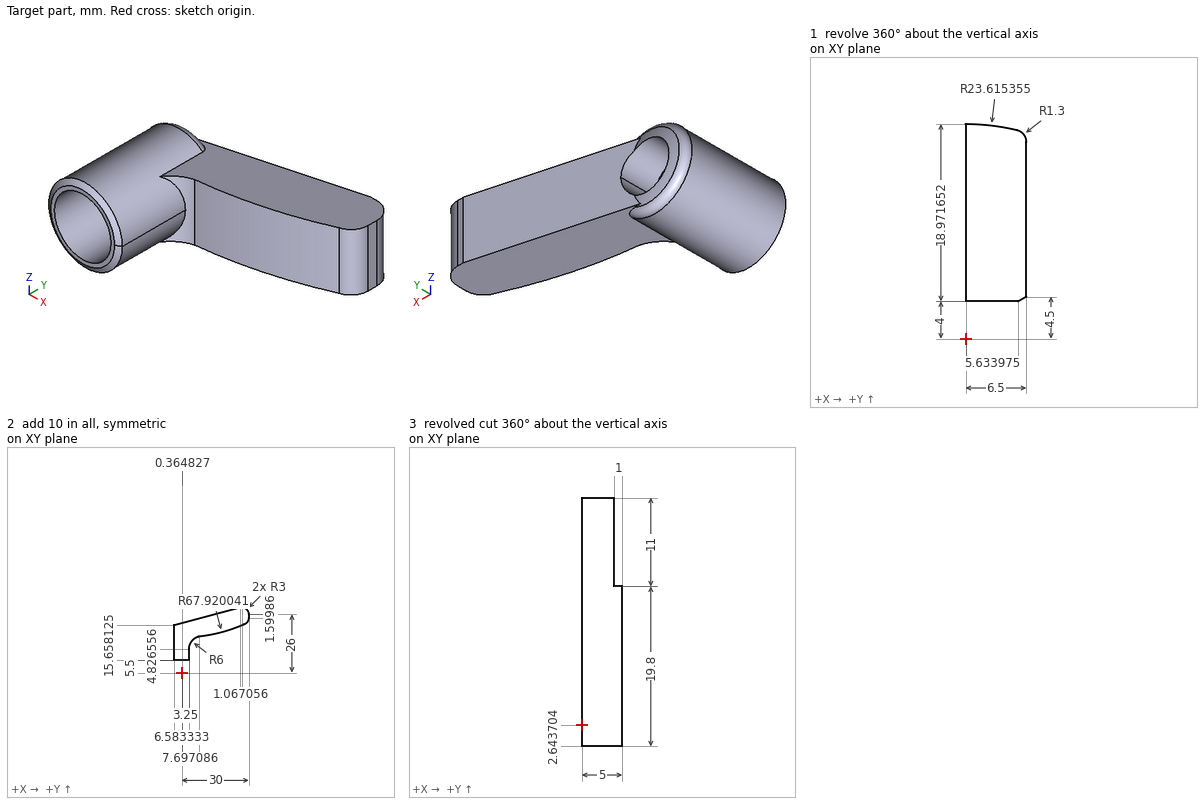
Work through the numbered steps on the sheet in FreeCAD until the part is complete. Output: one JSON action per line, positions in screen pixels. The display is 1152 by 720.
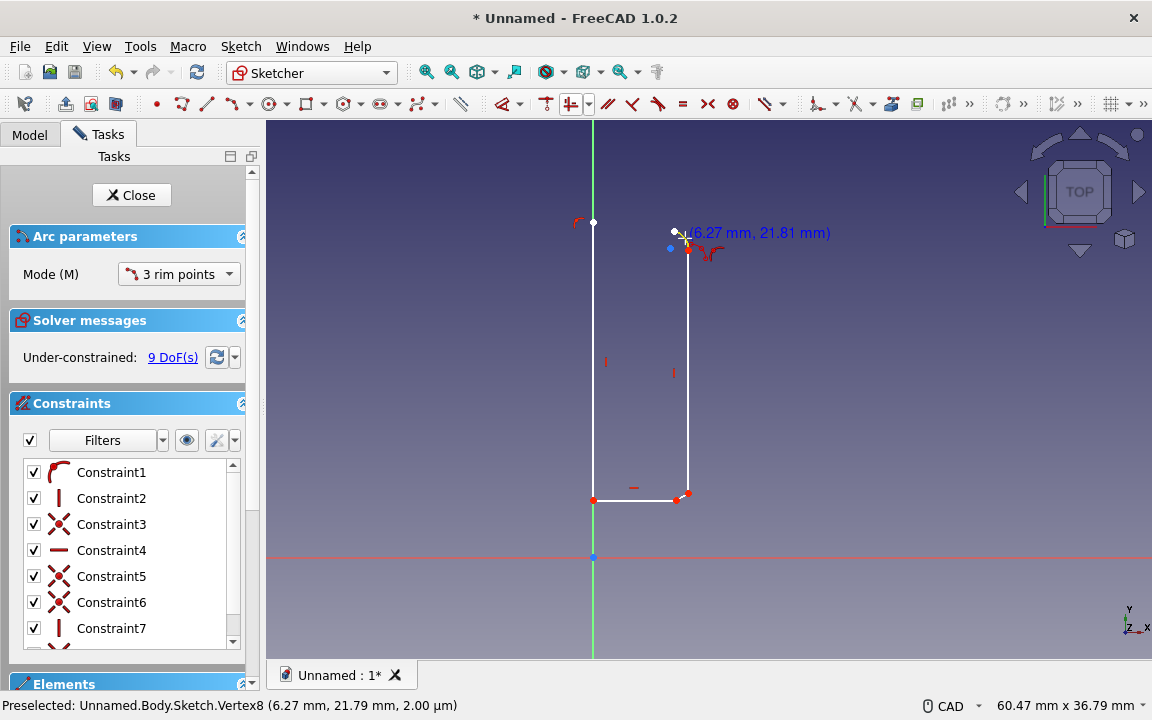
{"action": "left_click", "coordinate": [674, 232]}
{"action": "left_click", "coordinate": [593, 223]}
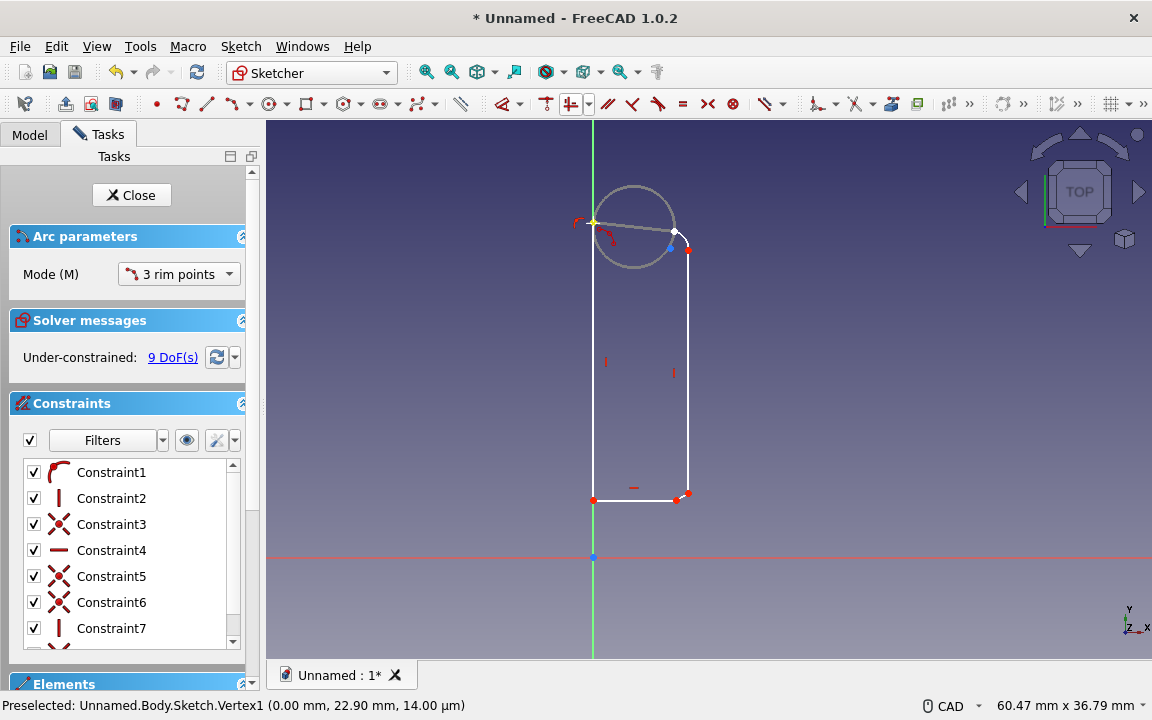
{"action": "scroll", "coordinate": [634, 224], "scroll_direction": "up", "scroll_amount": 10}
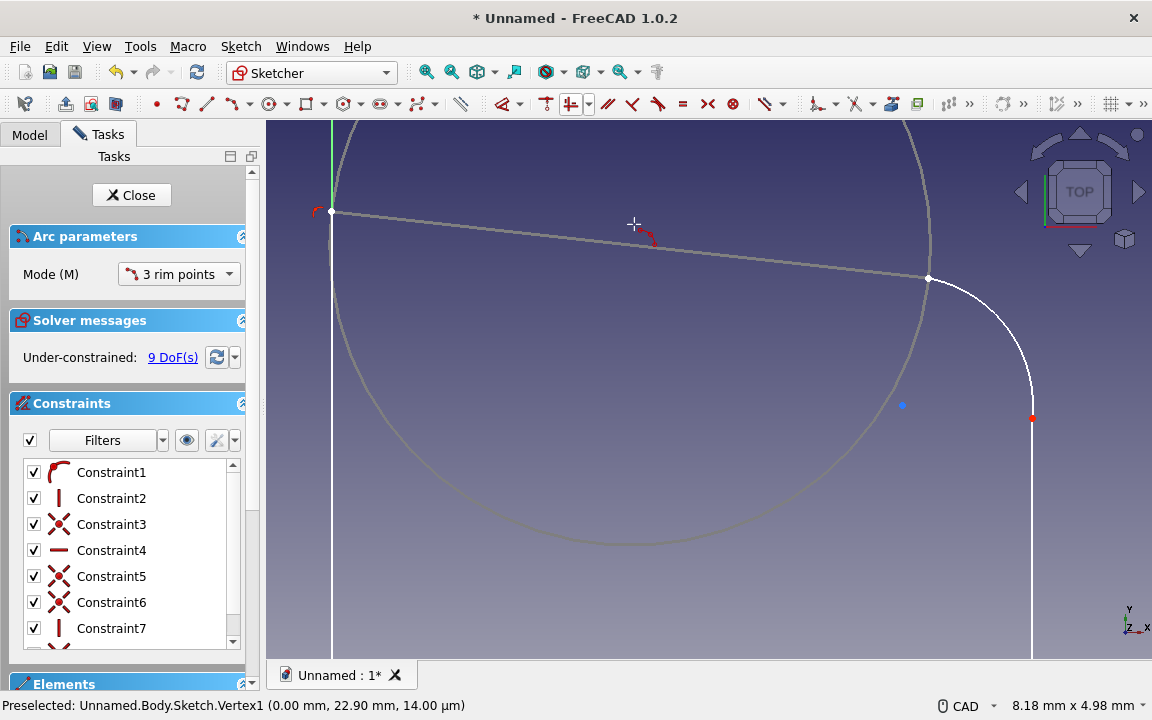
{"action": "left_click", "coordinate": [631, 221]}
{"action": "key", "text": "Escape"}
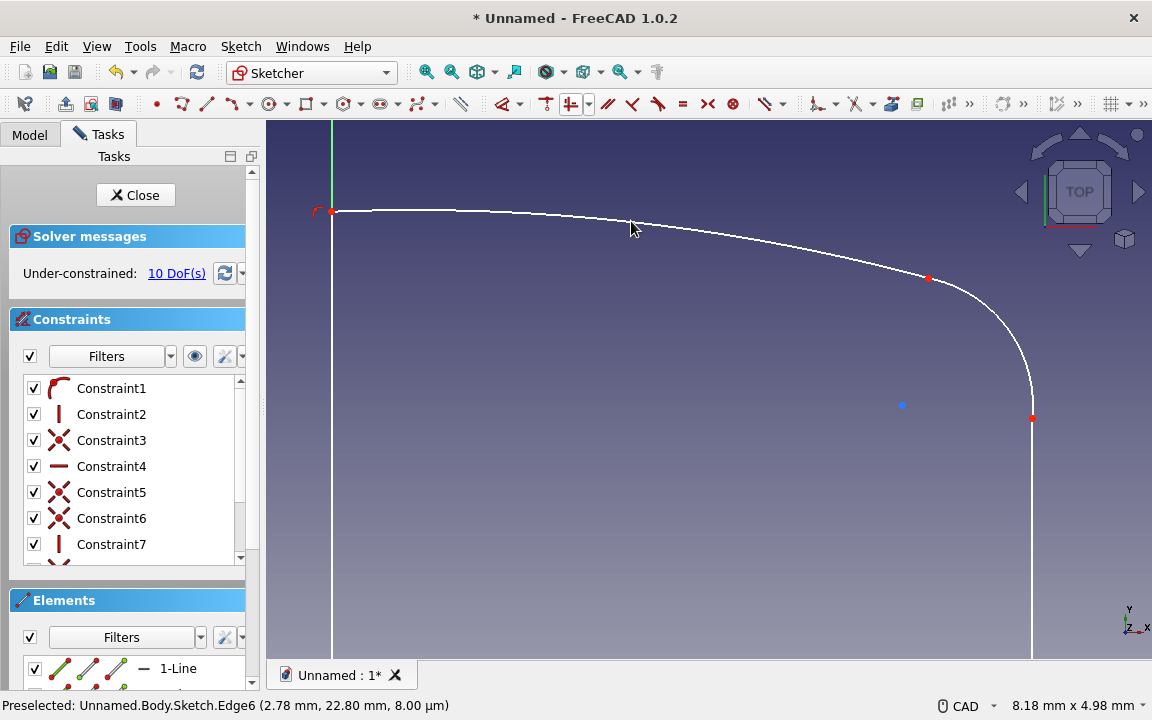
{"action": "scroll", "coordinate": [634, 224], "scroll_direction": "down", "scroll_amount": 10}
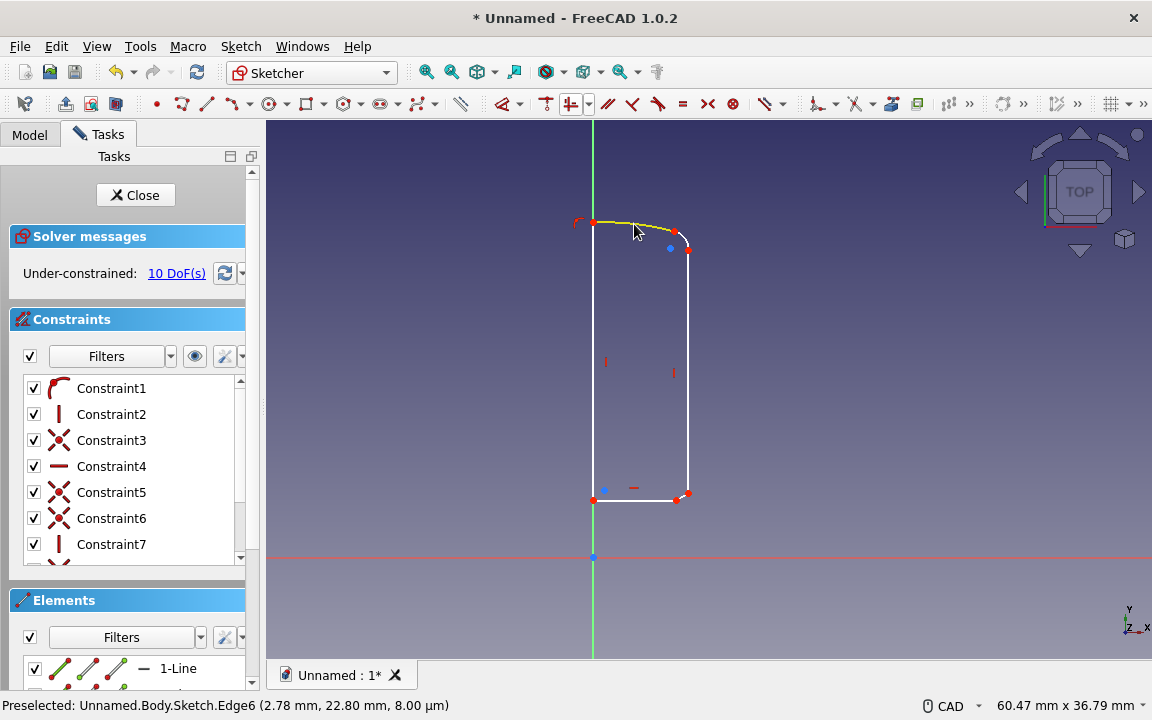
{"action": "left_click", "coordinate": [688, 421]}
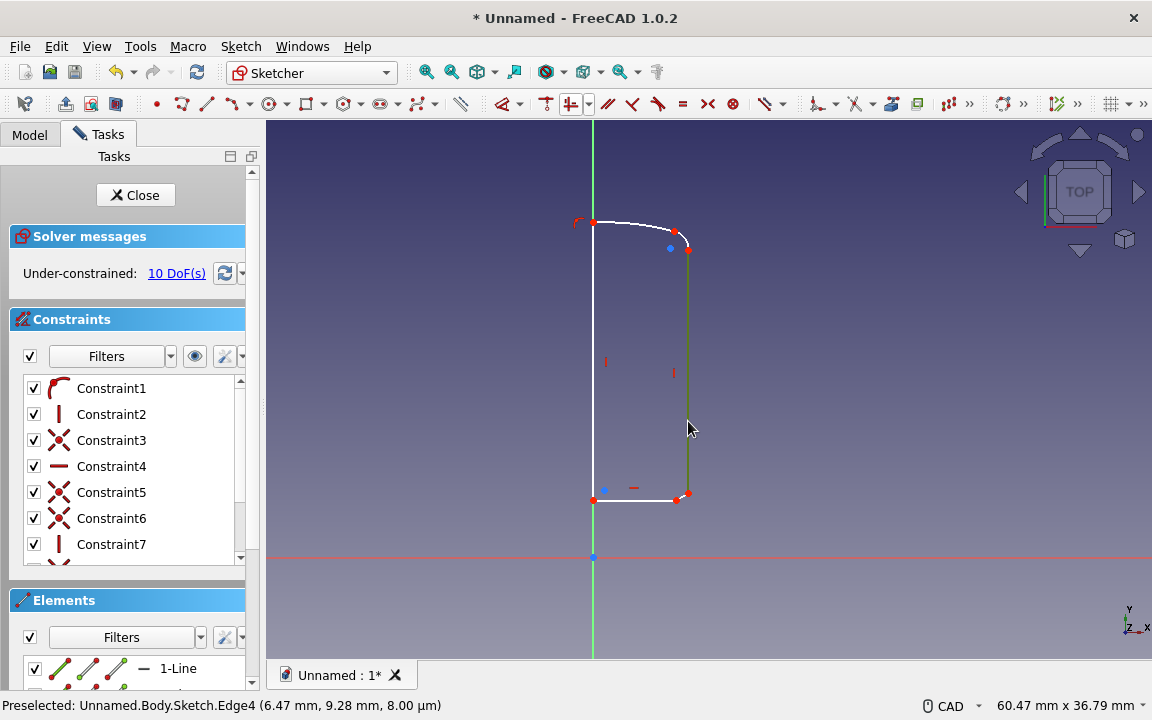
{"action": "left_click", "coordinate": [685, 238]}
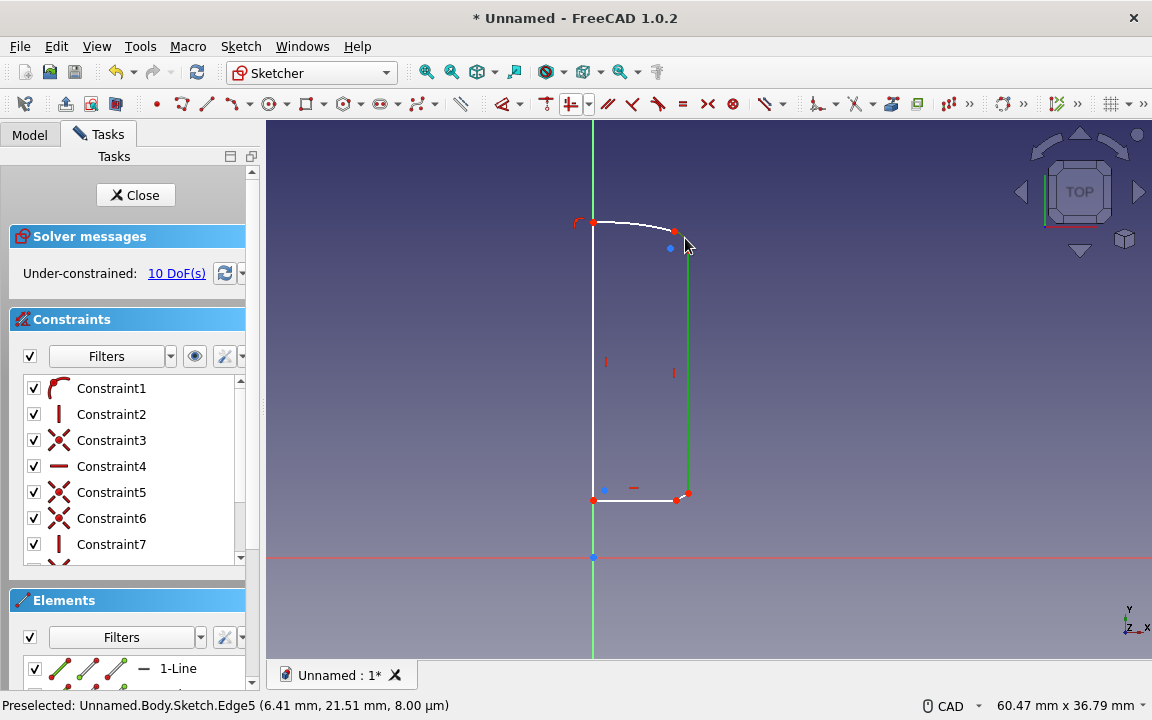
{"action": "key", "text": "t"}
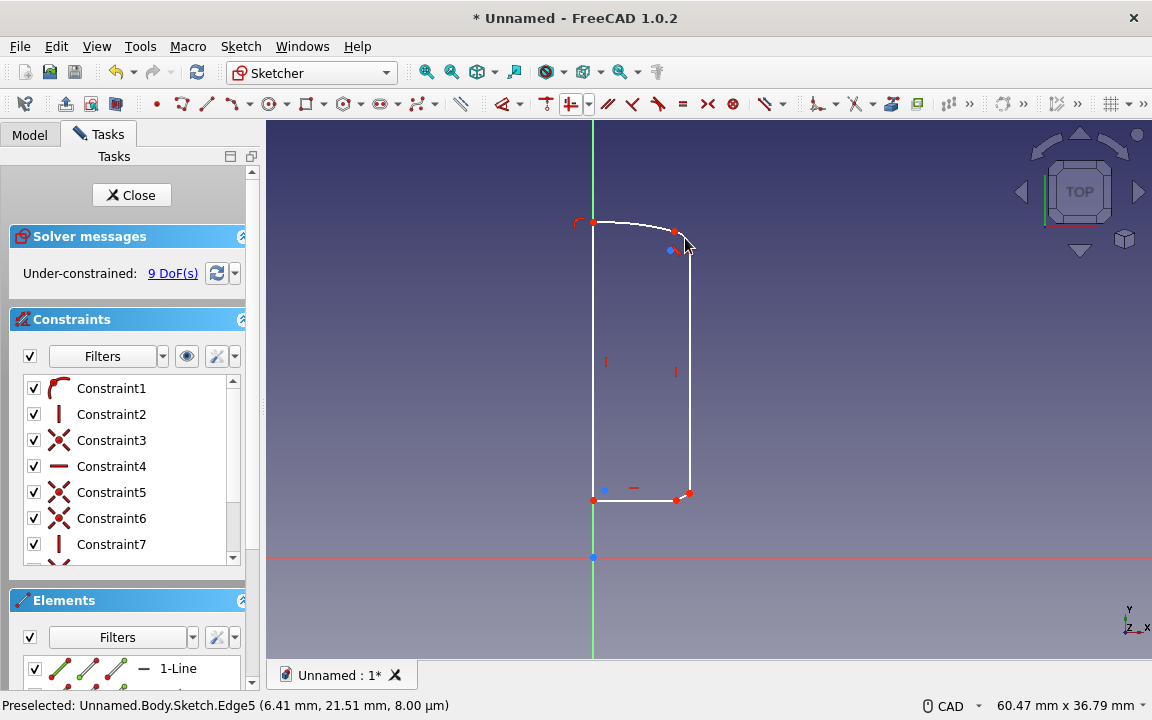
{"action": "left_click", "coordinate": [685, 238]}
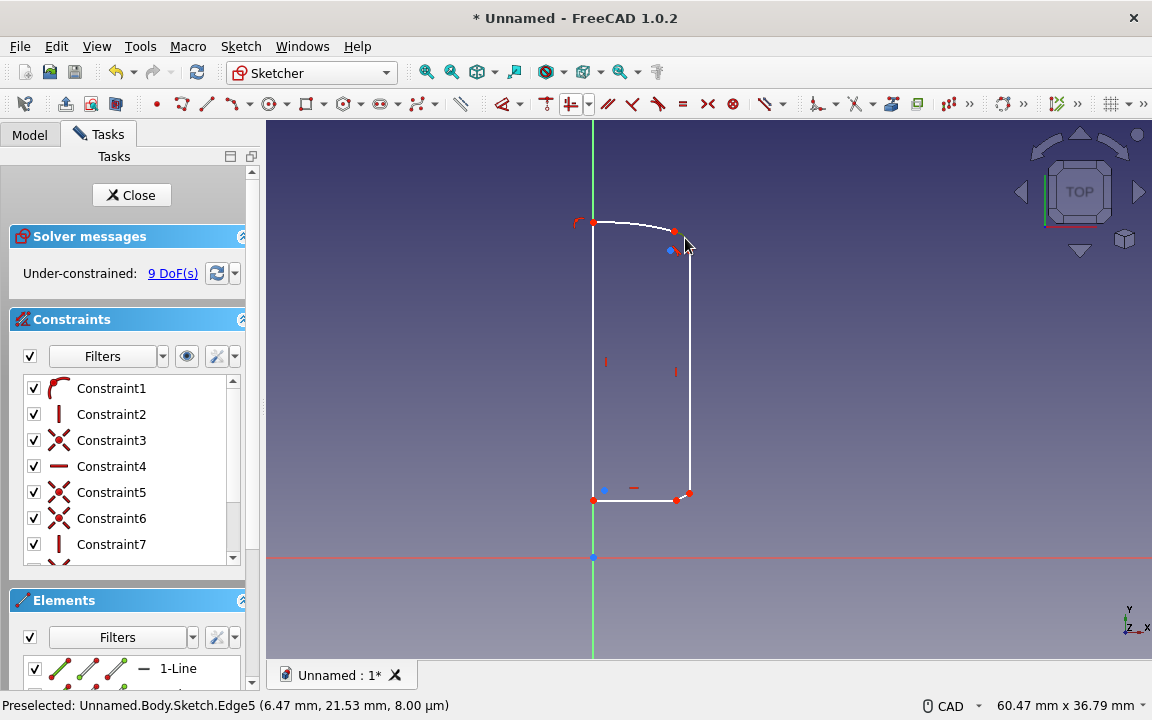
{"action": "left_click", "coordinate": [650, 226]}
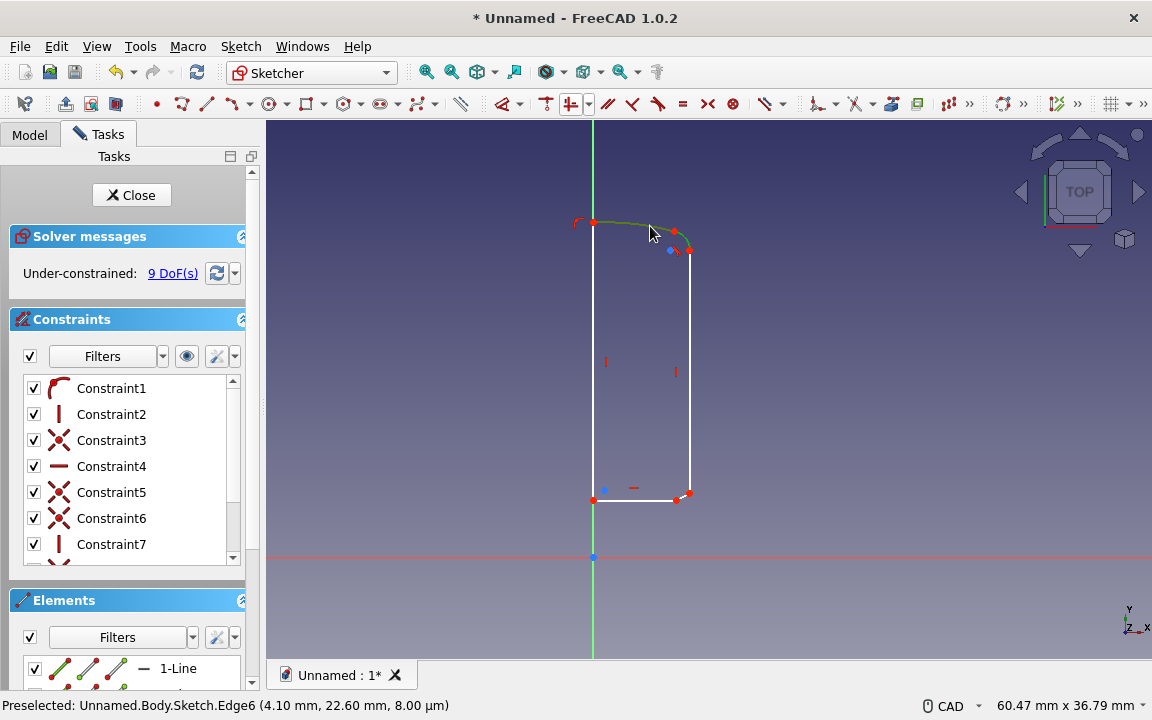
{"action": "key", "text": "t"}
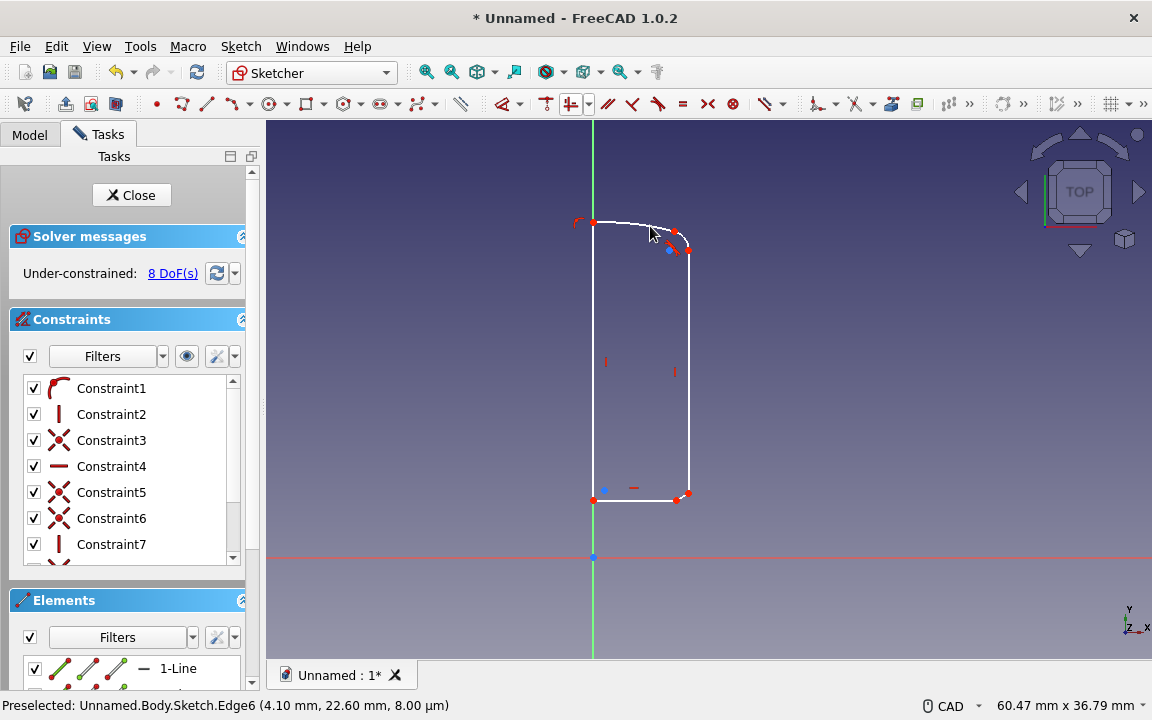
{"action": "left_click", "coordinate": [605, 490]}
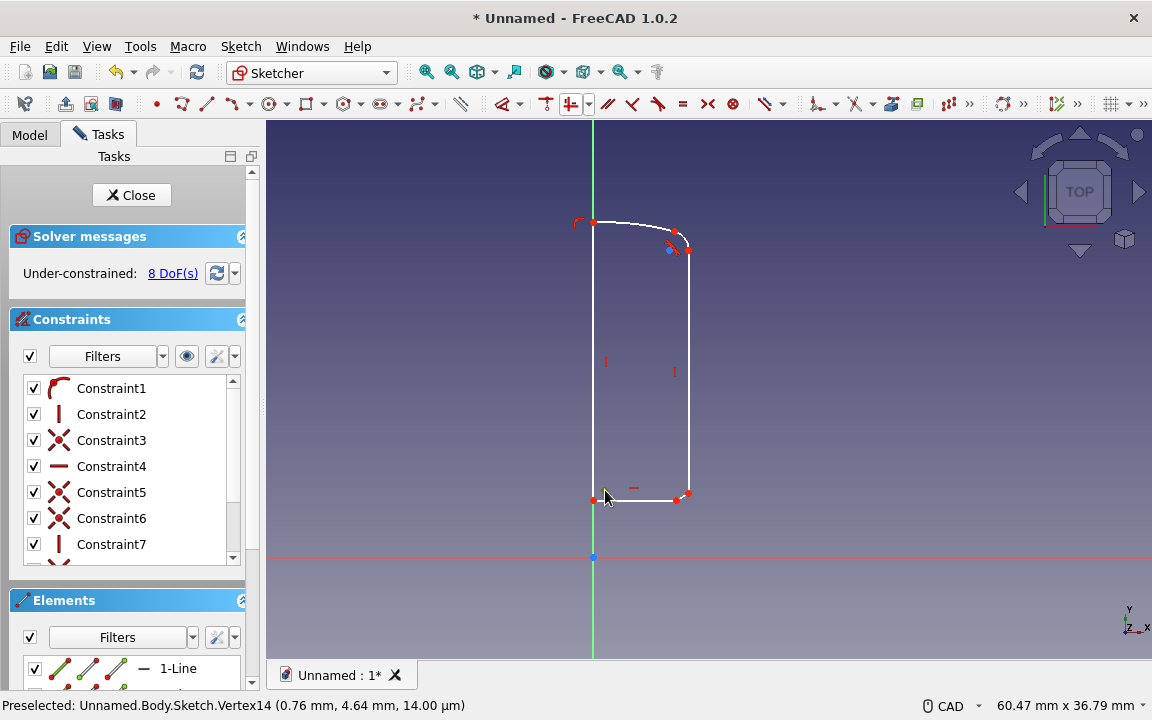
{"action": "left_click", "coordinate": [593, 596]}